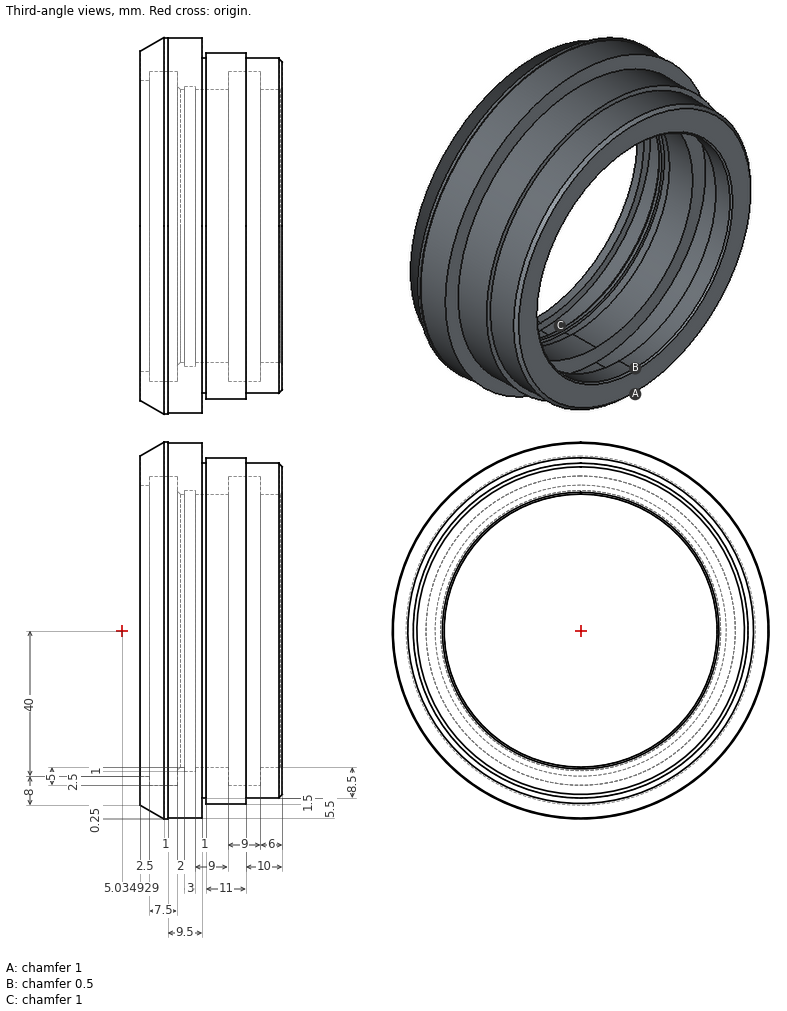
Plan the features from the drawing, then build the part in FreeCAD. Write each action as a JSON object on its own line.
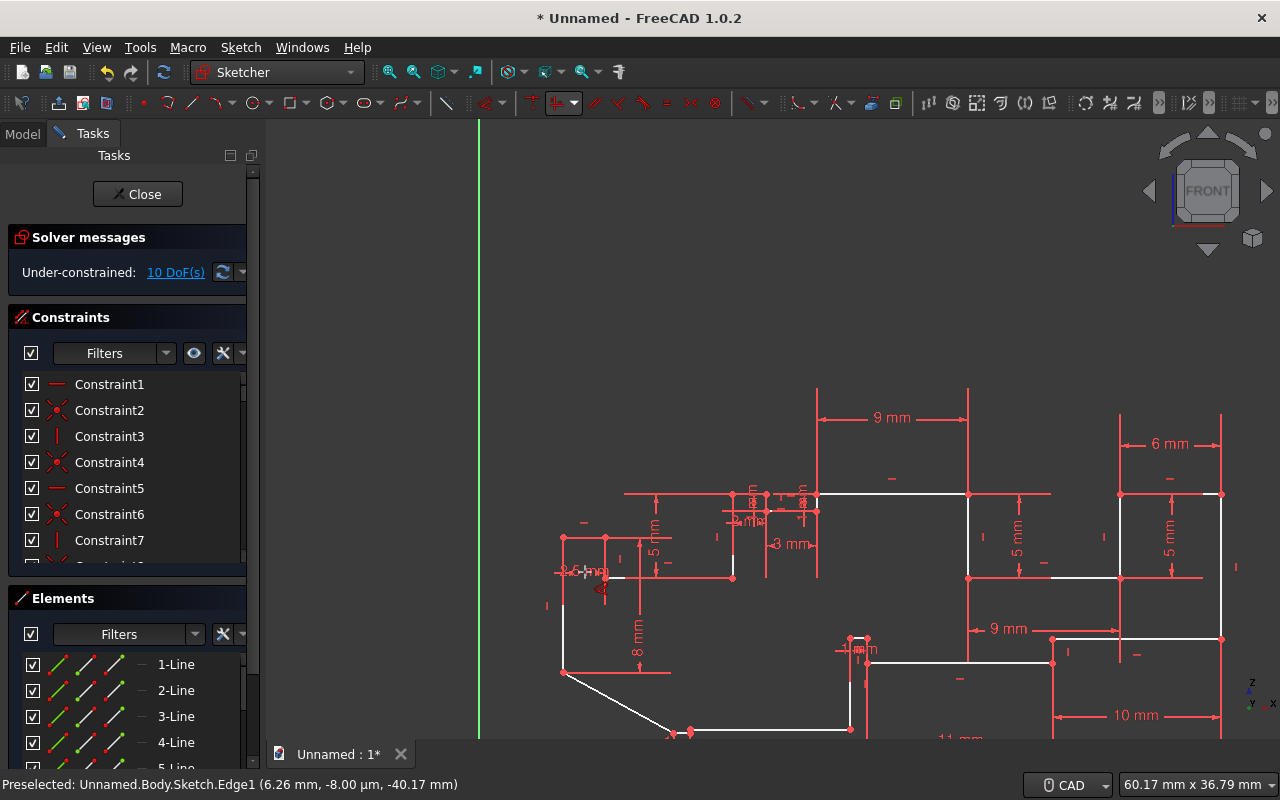
{"action": "left_click", "coordinate": [605, 550]}
{"action": "left_click", "coordinate": [547, 549]}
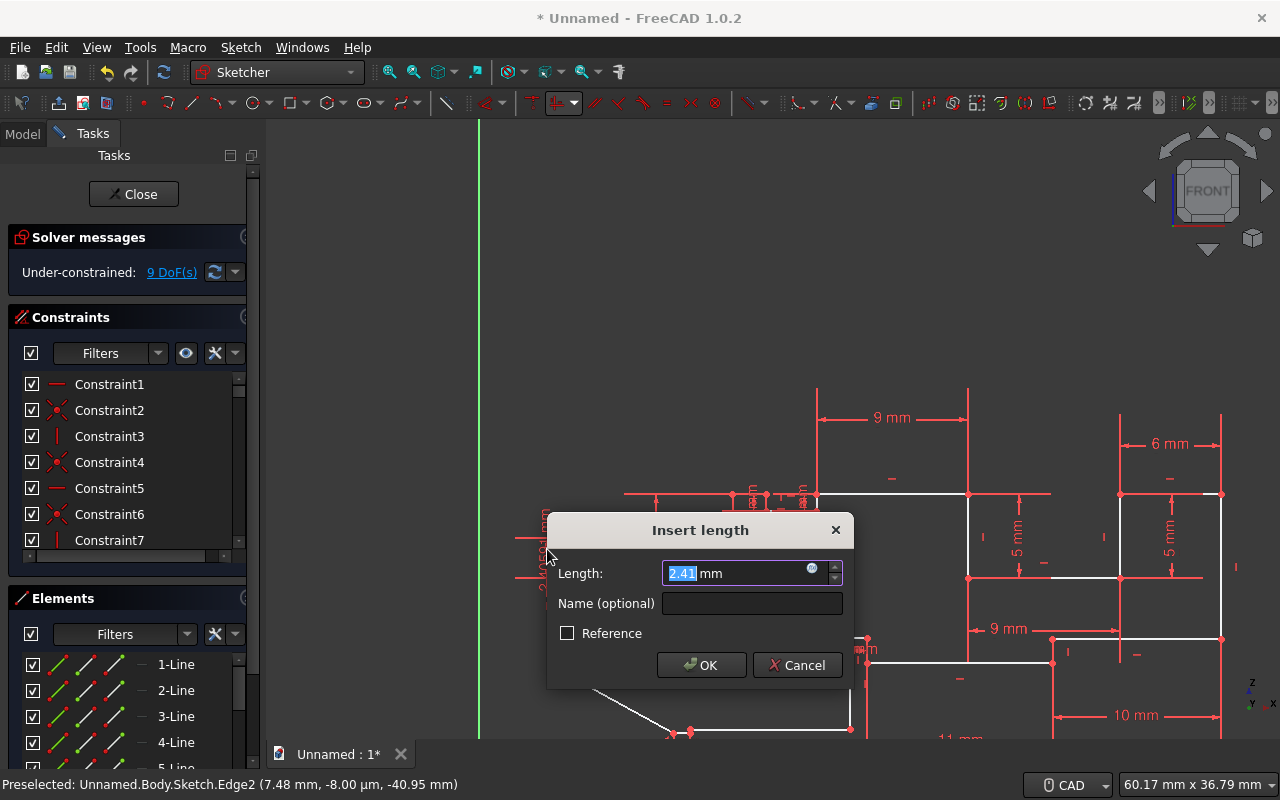
{"action": "type", "text": "2.5"}
{"action": "key", "text": "Return"}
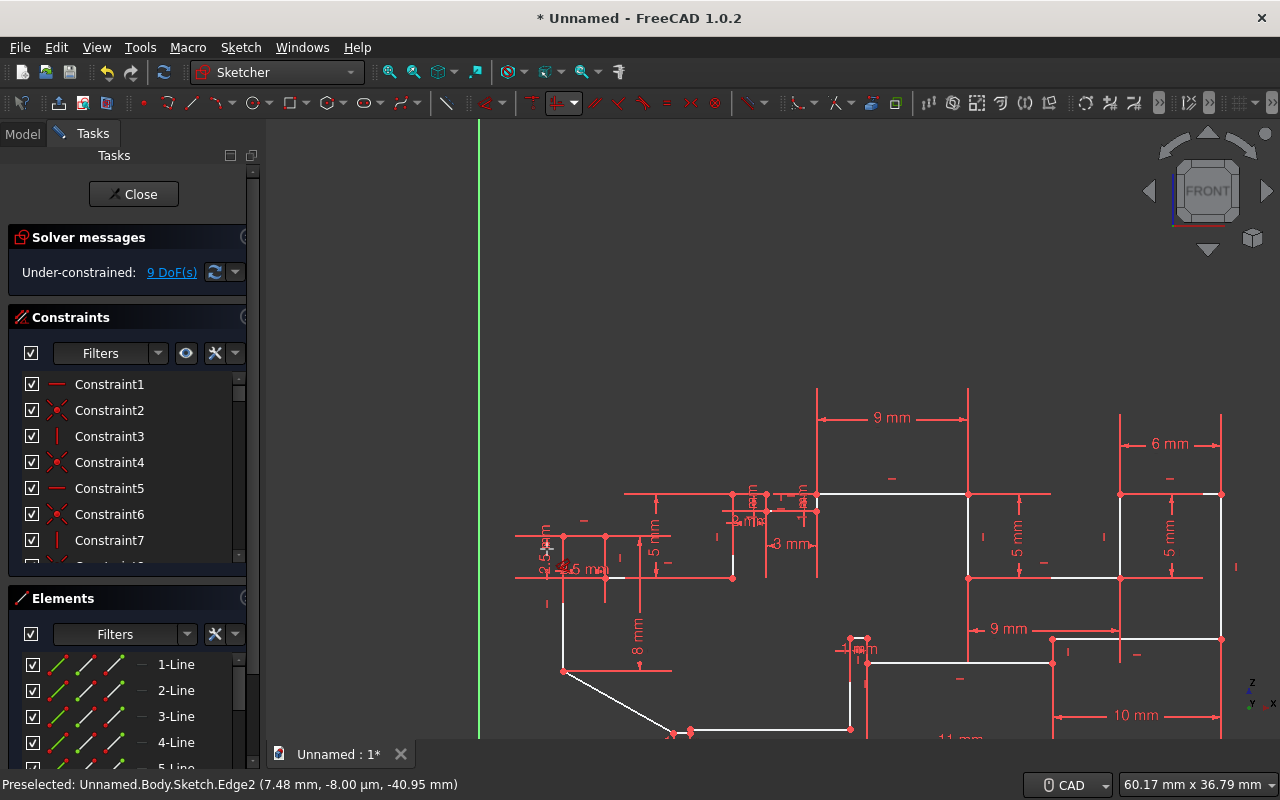
{"action": "left_click", "coordinate": [644, 578]}
{"action": "left_click", "coordinate": [669, 612]}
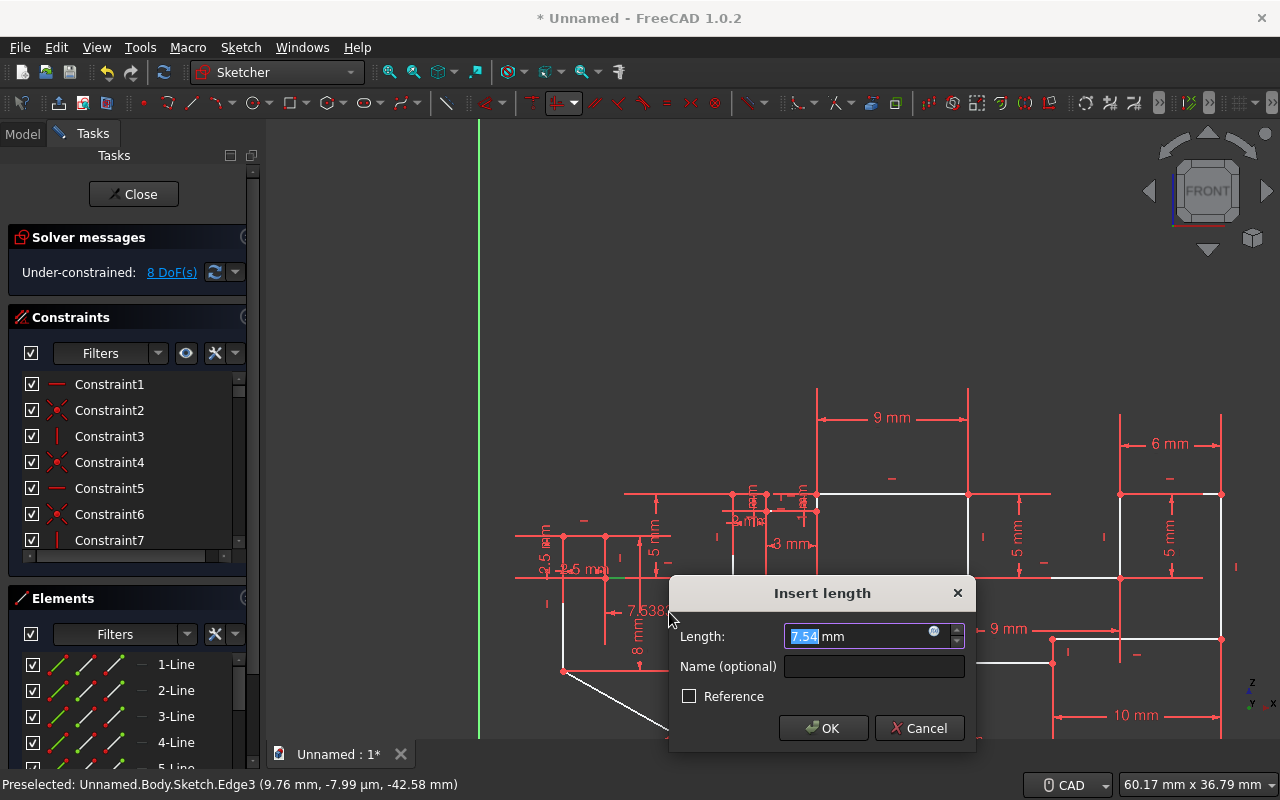
{"action": "type", "text": "7.5"}
{"action": "key", "text": "Return"}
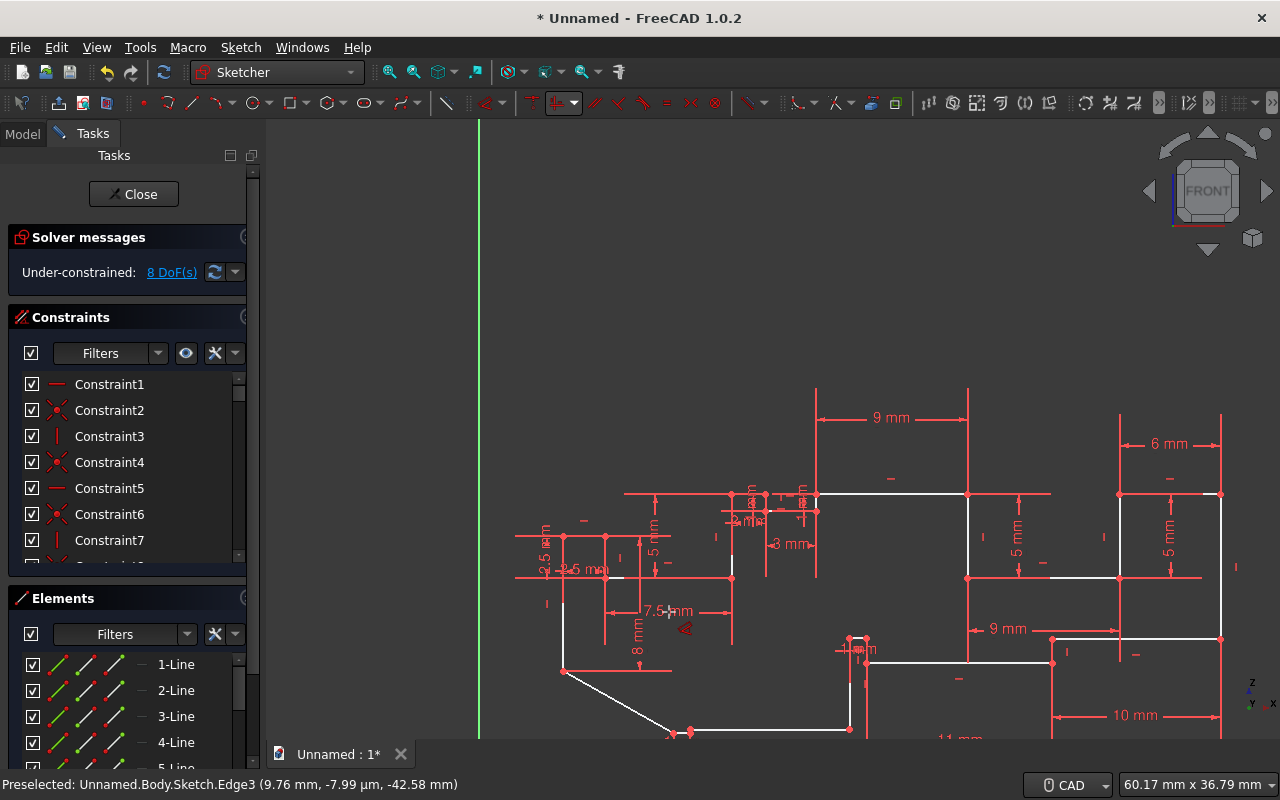
{"action": "scroll", "coordinate": [585, 537], "scroll_direction": "down", "scroll_amount": 4}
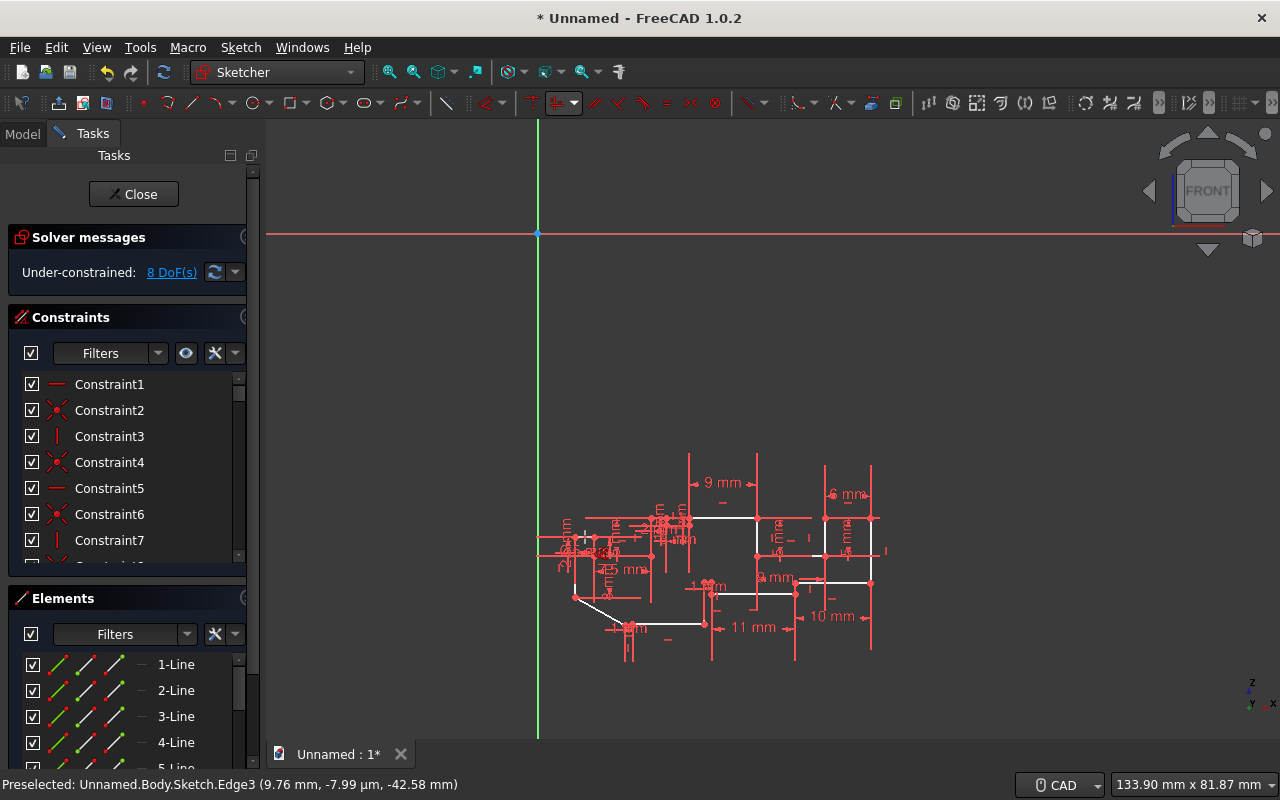
{"action": "left_click", "coordinate": [871, 538]}
{"action": "left_click", "coordinate": [905, 566]}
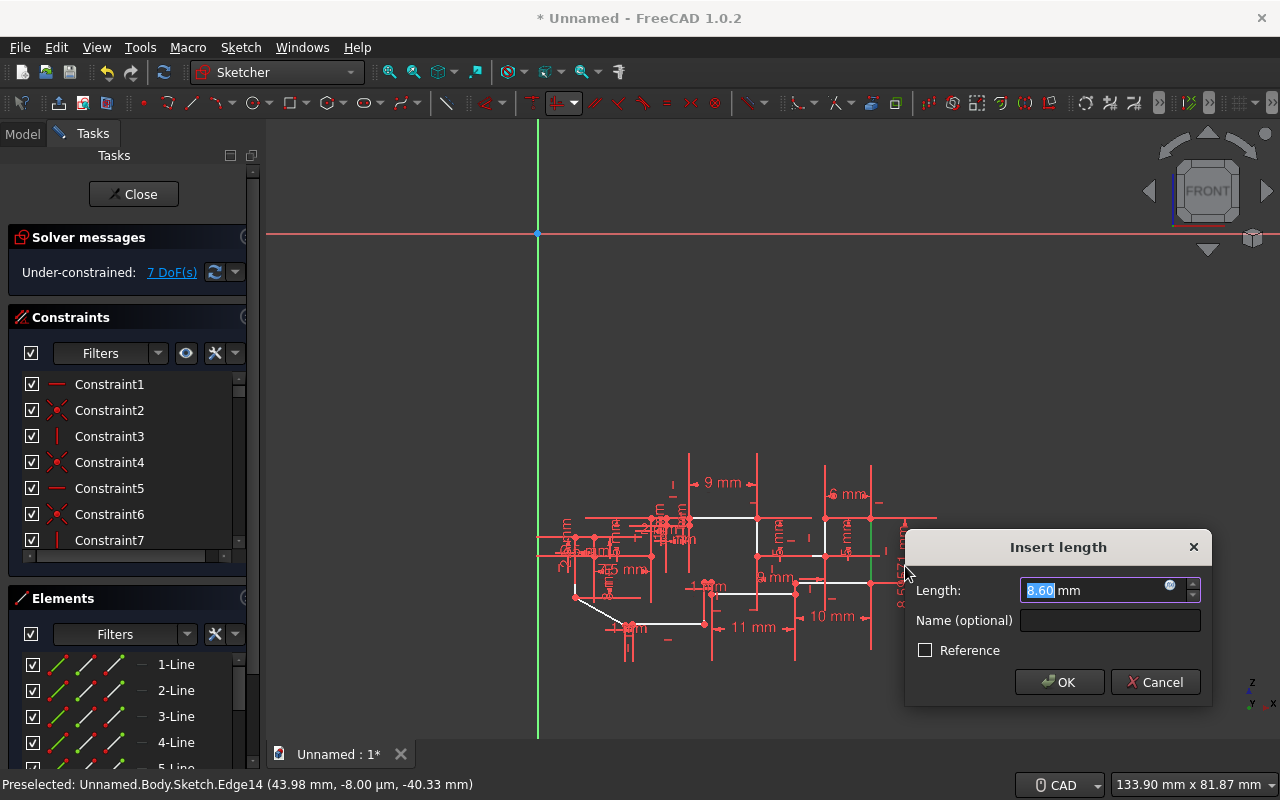
{"action": "type", "text": "8.5"}
{"action": "key", "text": "Return"}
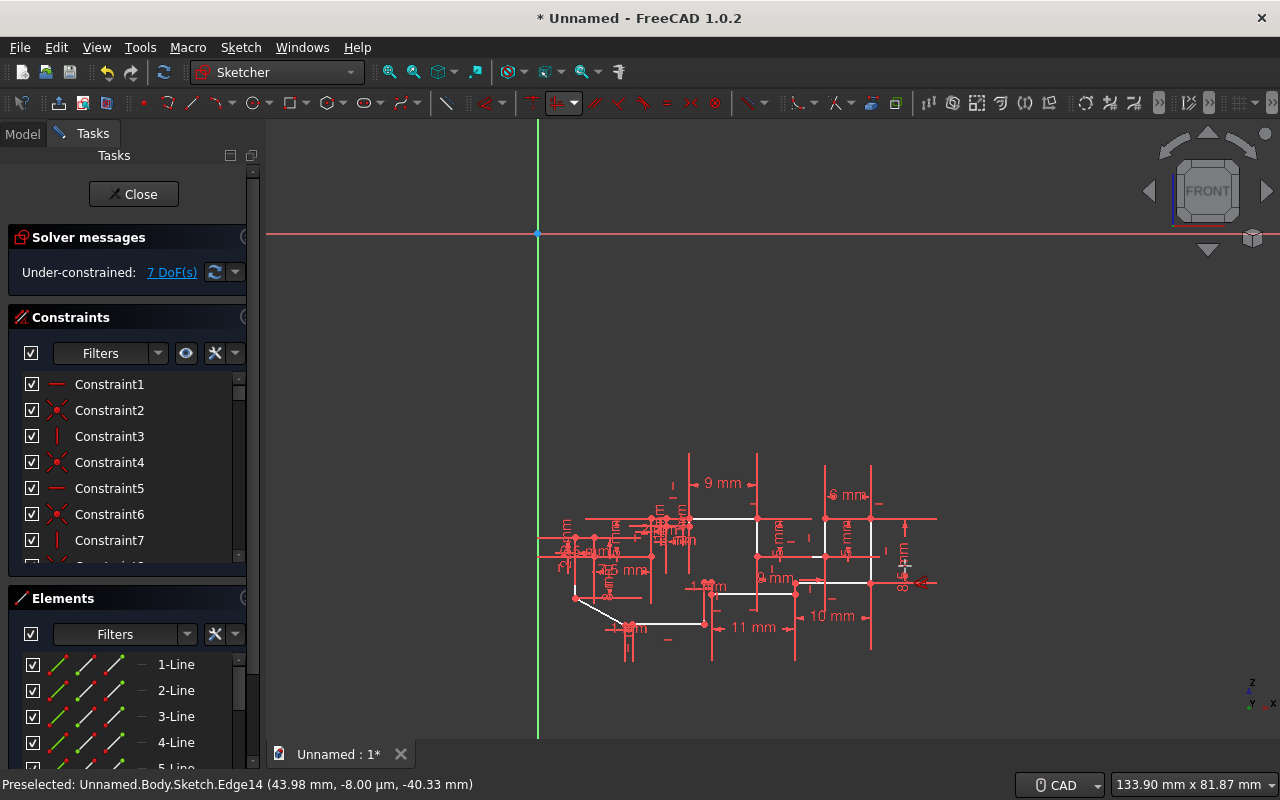
{"action": "scroll", "coordinate": [795, 589], "scroll_direction": "up", "scroll_amount": 7}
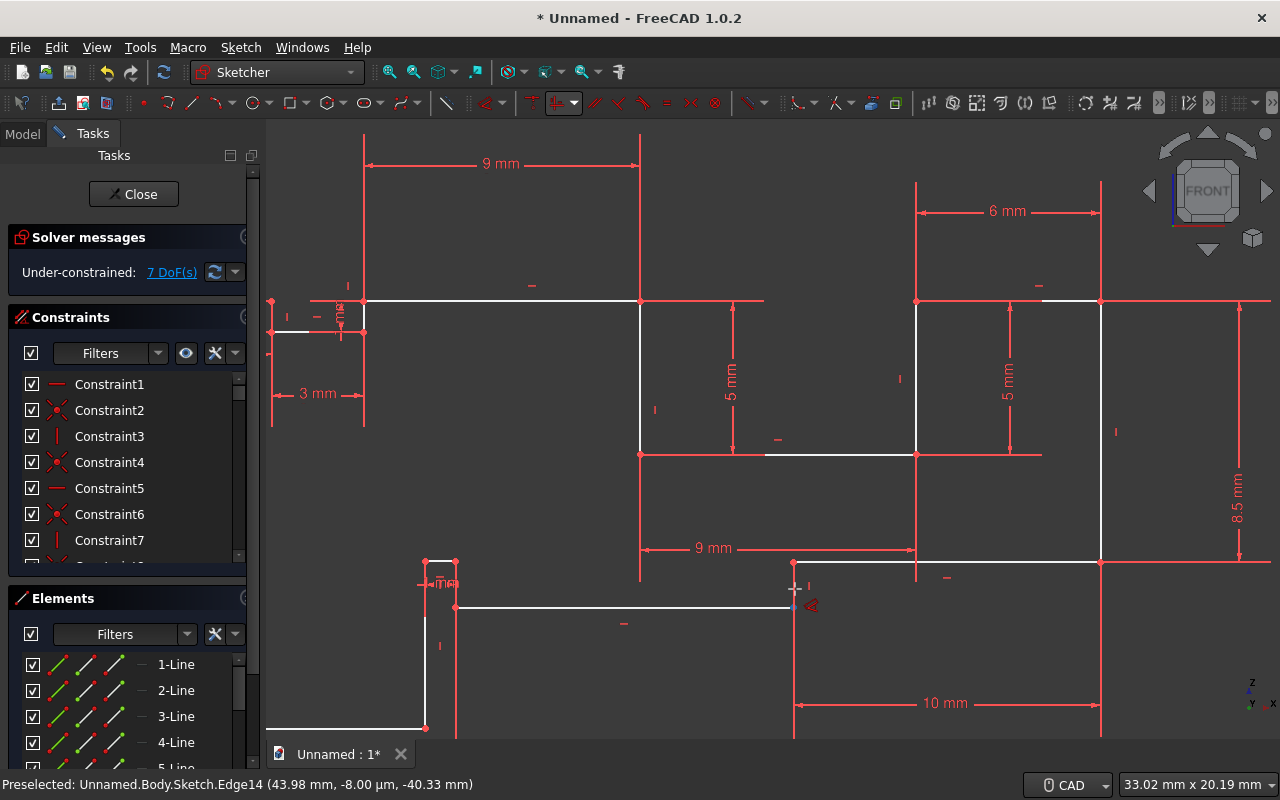
{"action": "left_click", "coordinate": [794, 585]}
{"action": "left_click", "coordinate": [828, 585]}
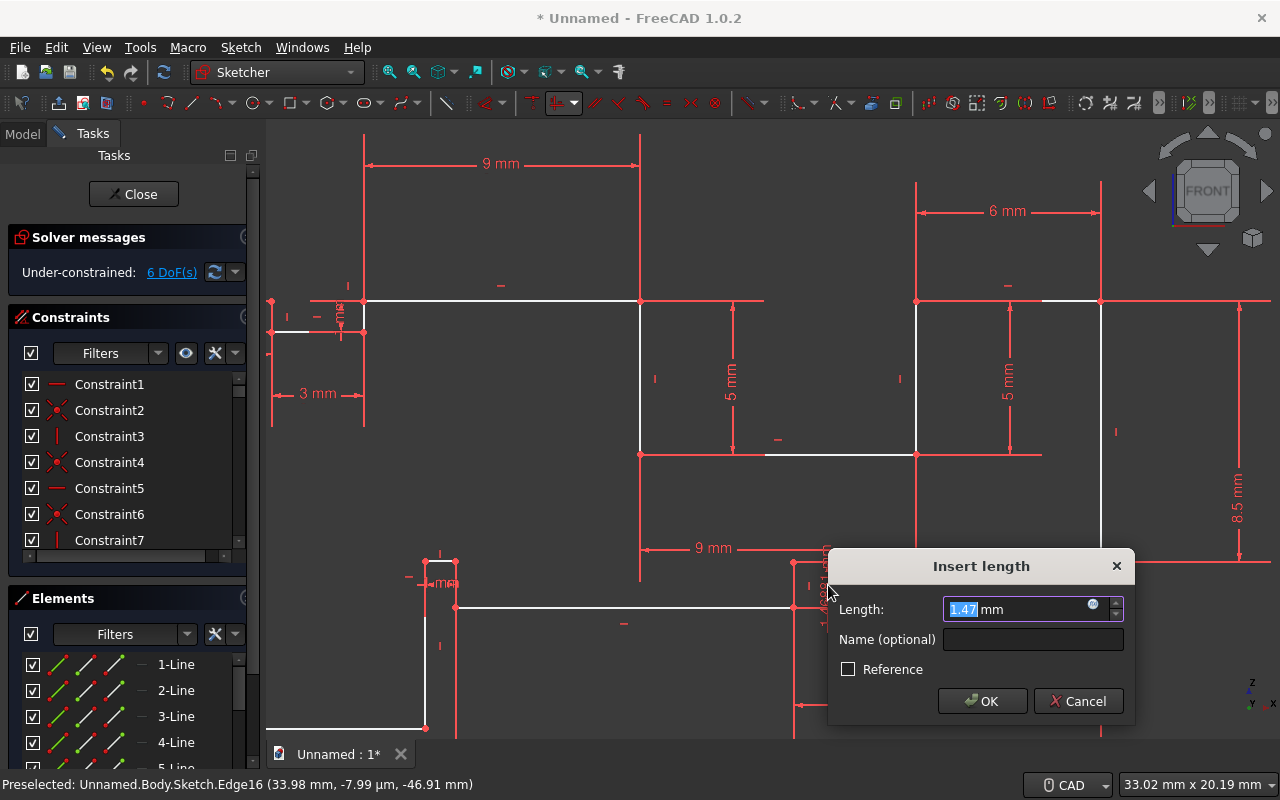
{"action": "type", "text": "1.5"}
{"action": "key", "text": "Return"}